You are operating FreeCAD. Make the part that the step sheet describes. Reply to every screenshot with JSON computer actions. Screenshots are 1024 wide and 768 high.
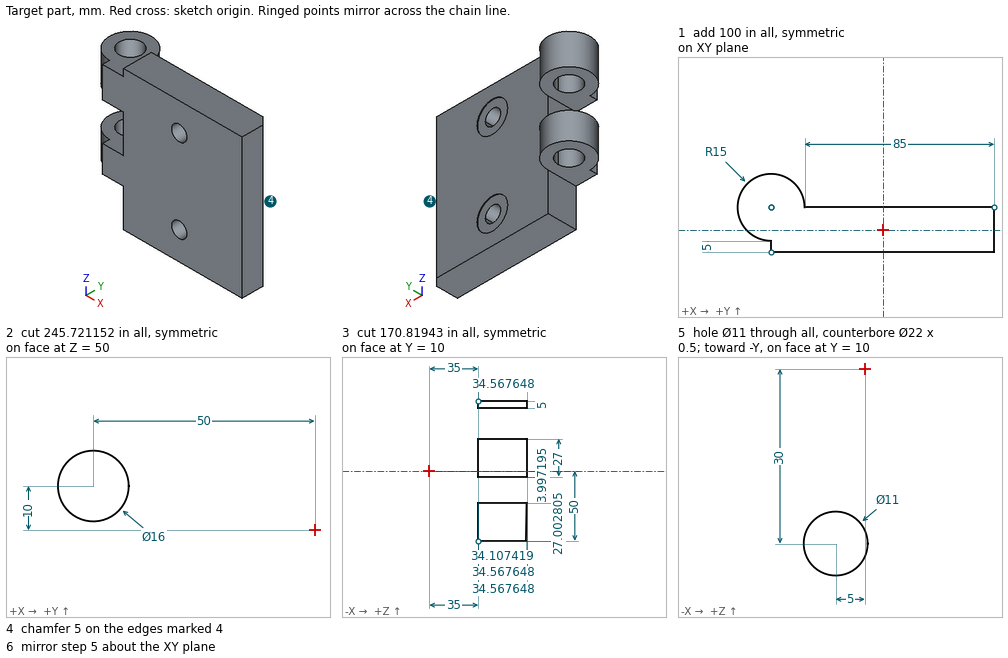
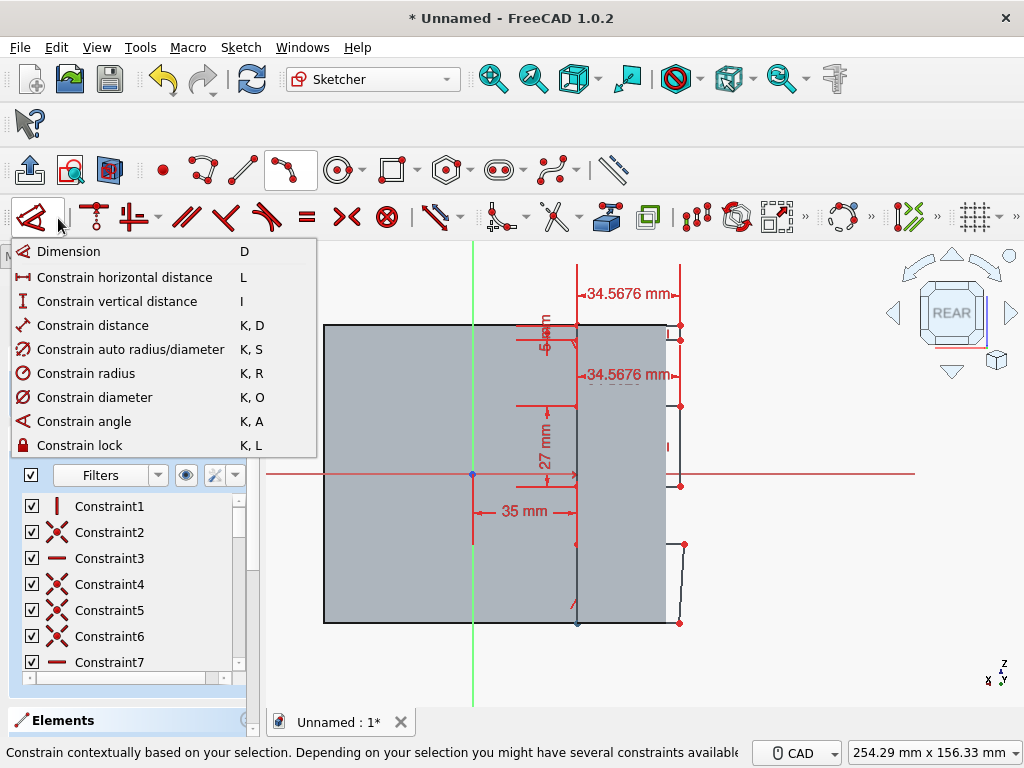
{"action": "left_click", "coordinate": [164, 301]}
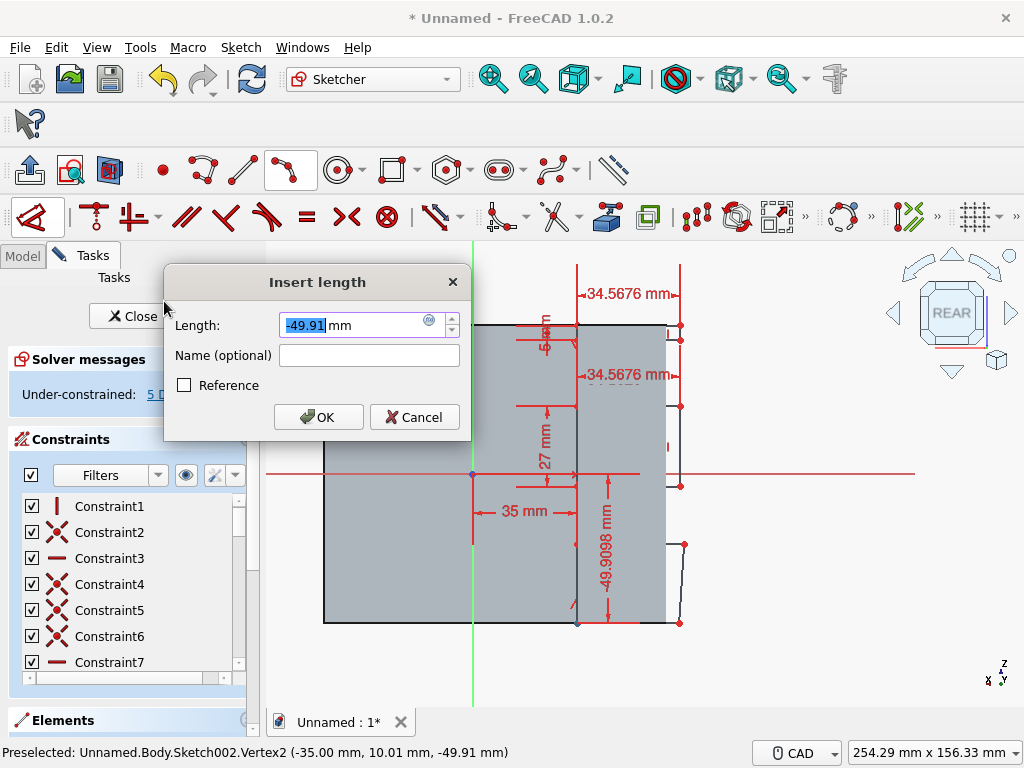
{"action": "type", "text": "-50"}
{"action": "key", "text": "Return"}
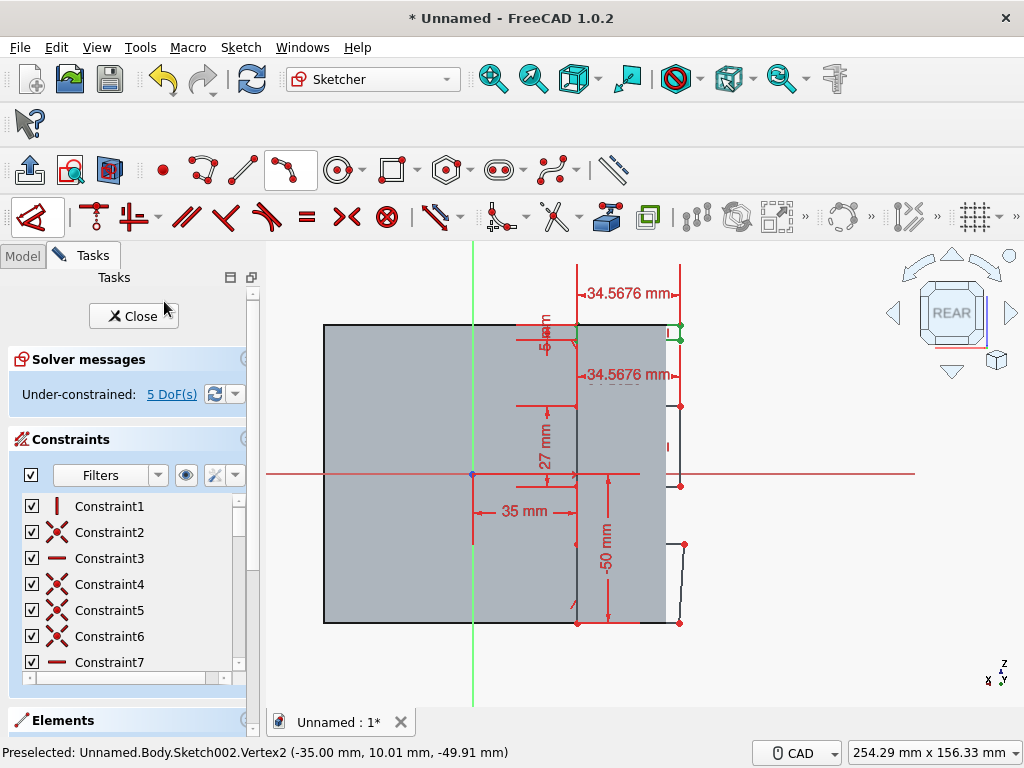
{"action": "left_click", "coordinate": [577, 406]}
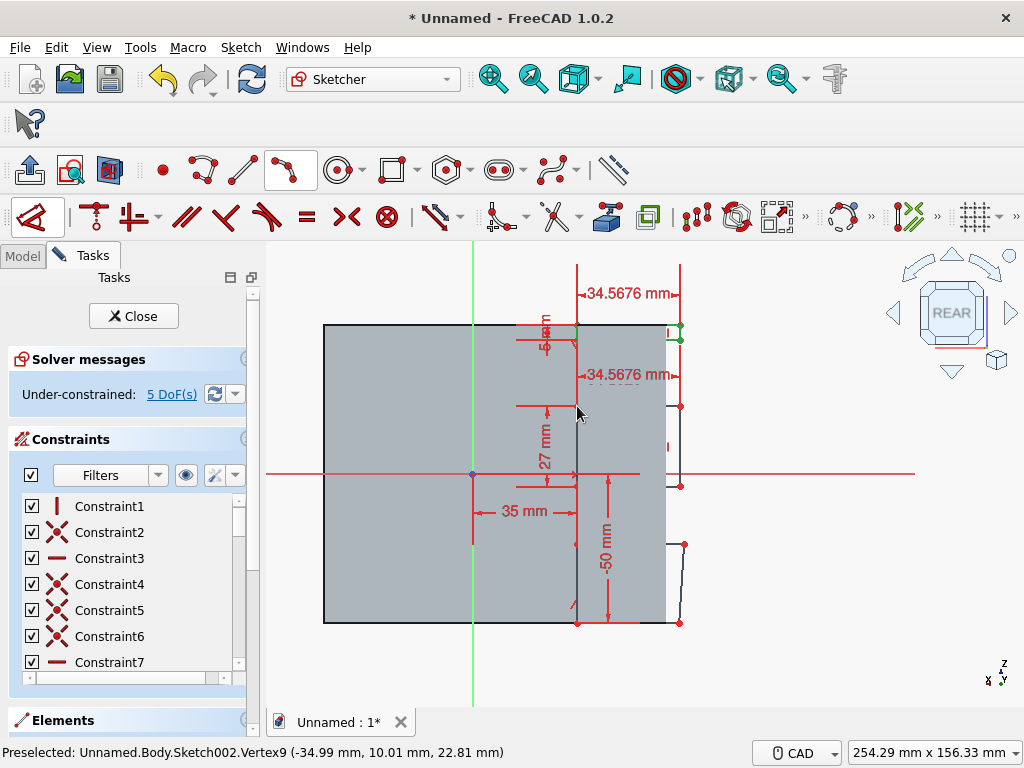
{"action": "key", "text": "l"}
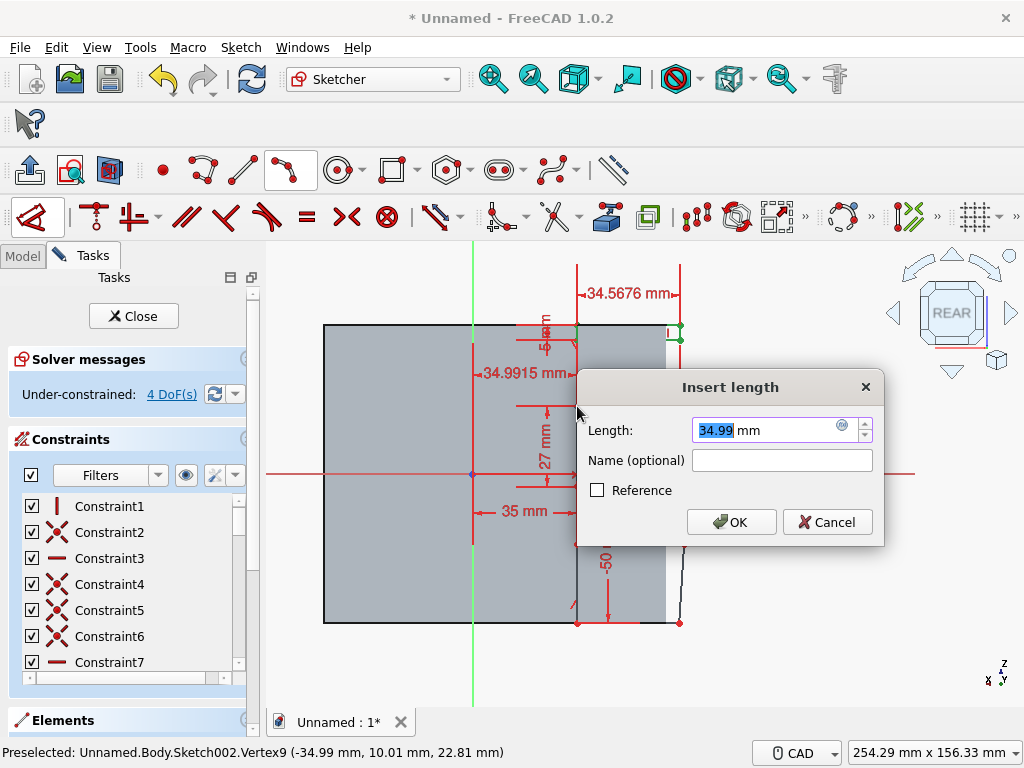
{"action": "type", "text": "35"}
{"action": "key", "text": "Return"}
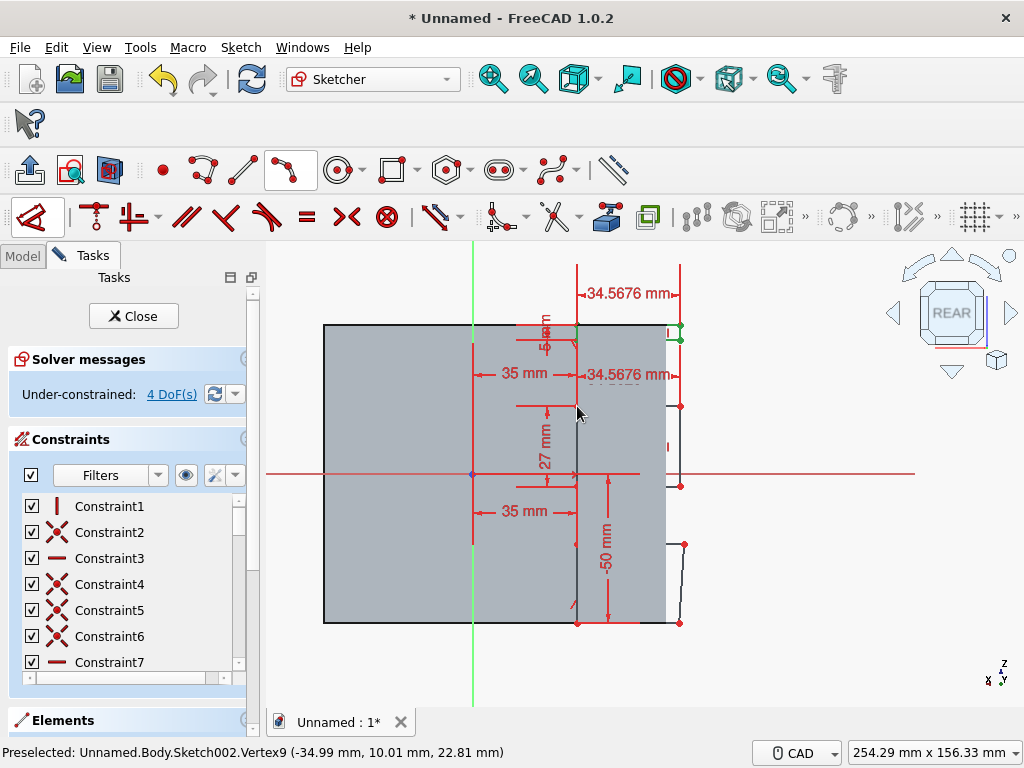
{"action": "left_click", "coordinate": [577, 568]}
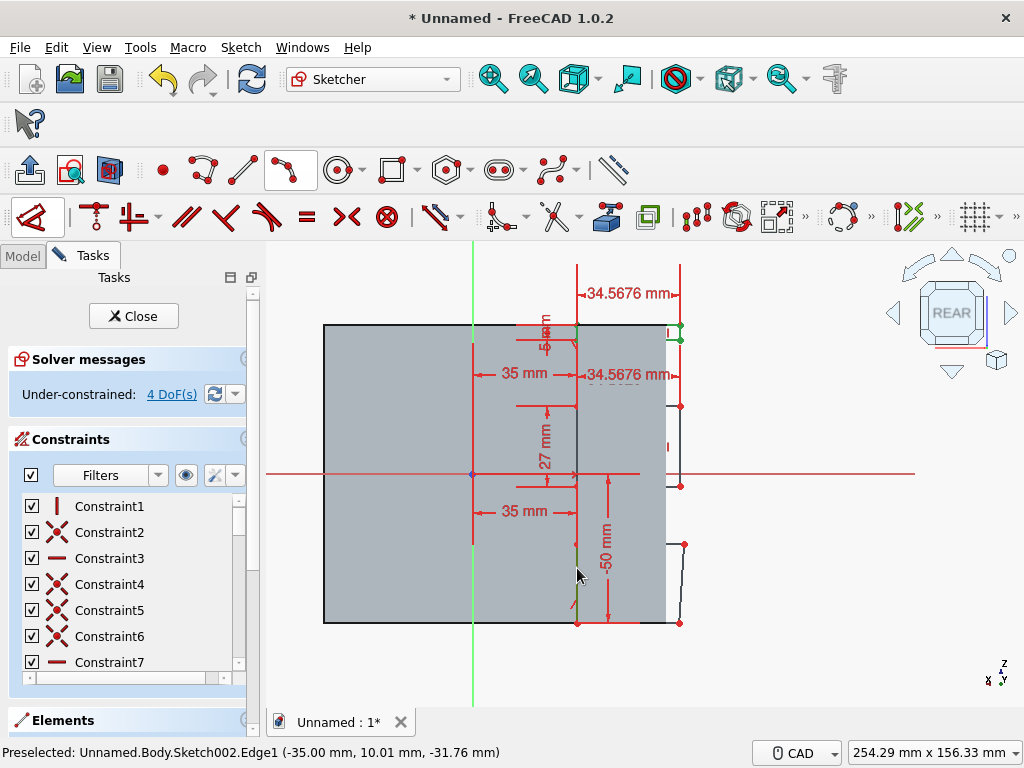
{"action": "key", "text": "i"}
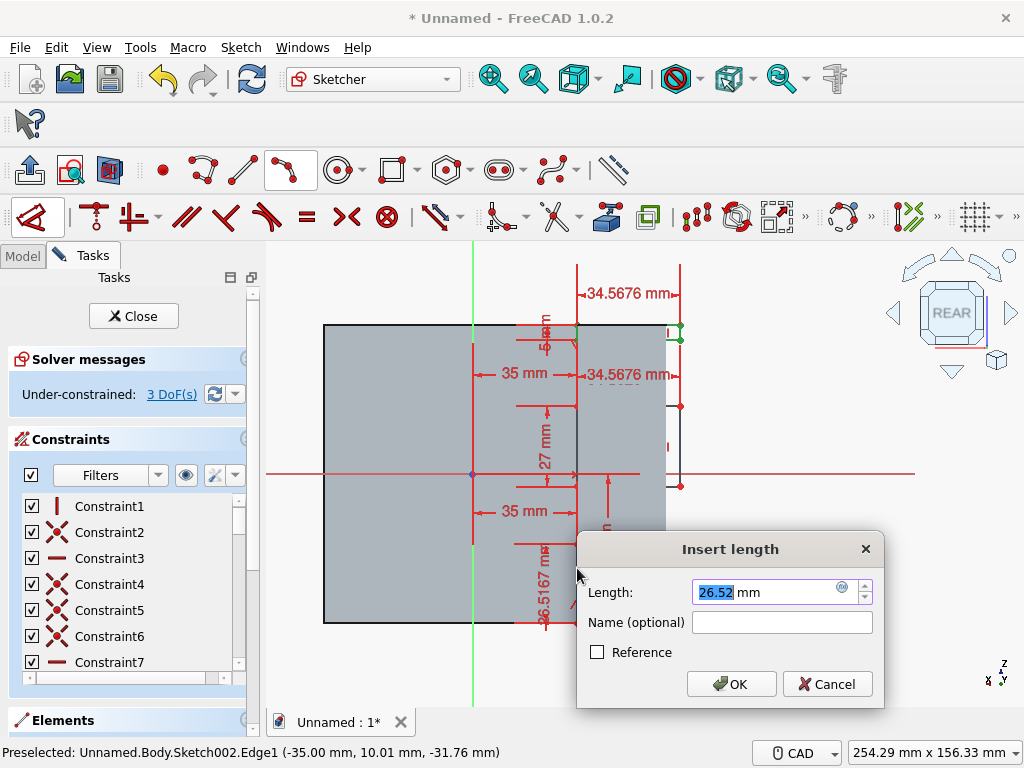
{"action": "type", "text": "27.002805"}
{"action": "key", "text": "Return"}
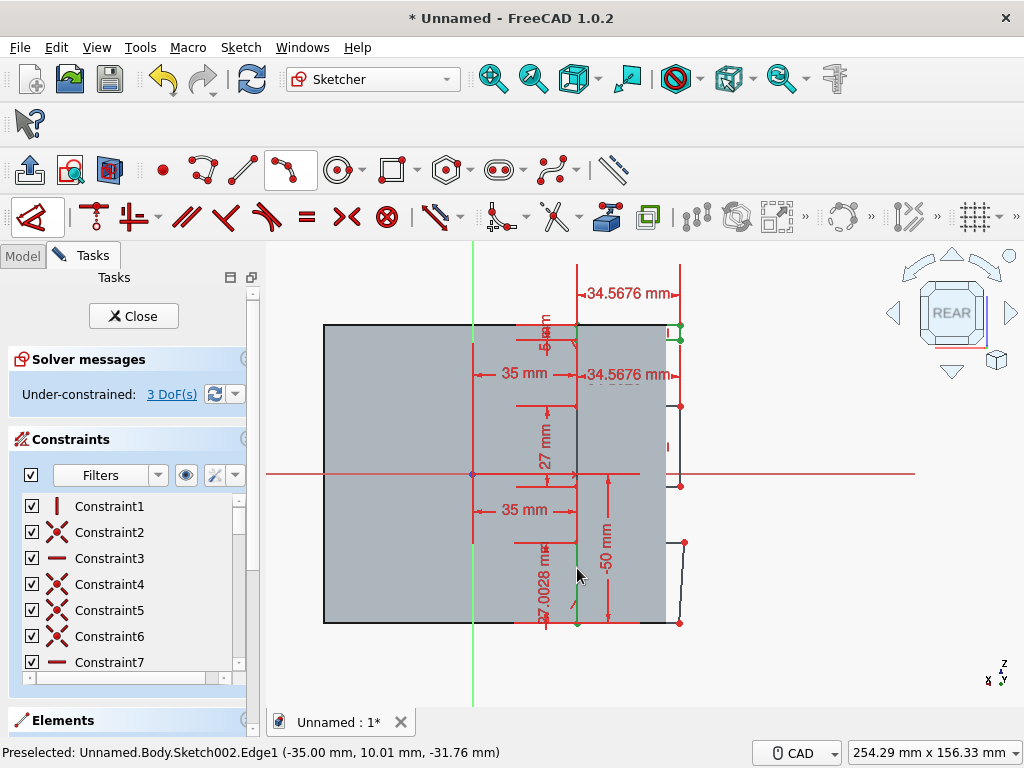
{"action": "left_click", "coordinate": [608, 623]}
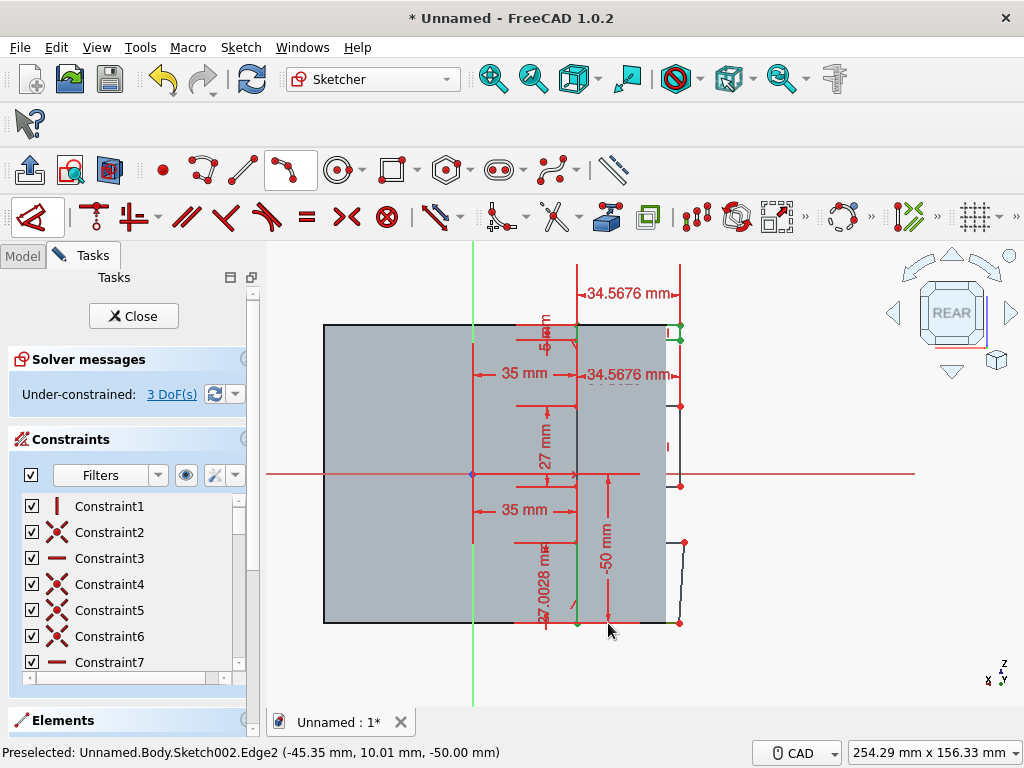
{"action": "left_click", "coordinate": [58, 218]}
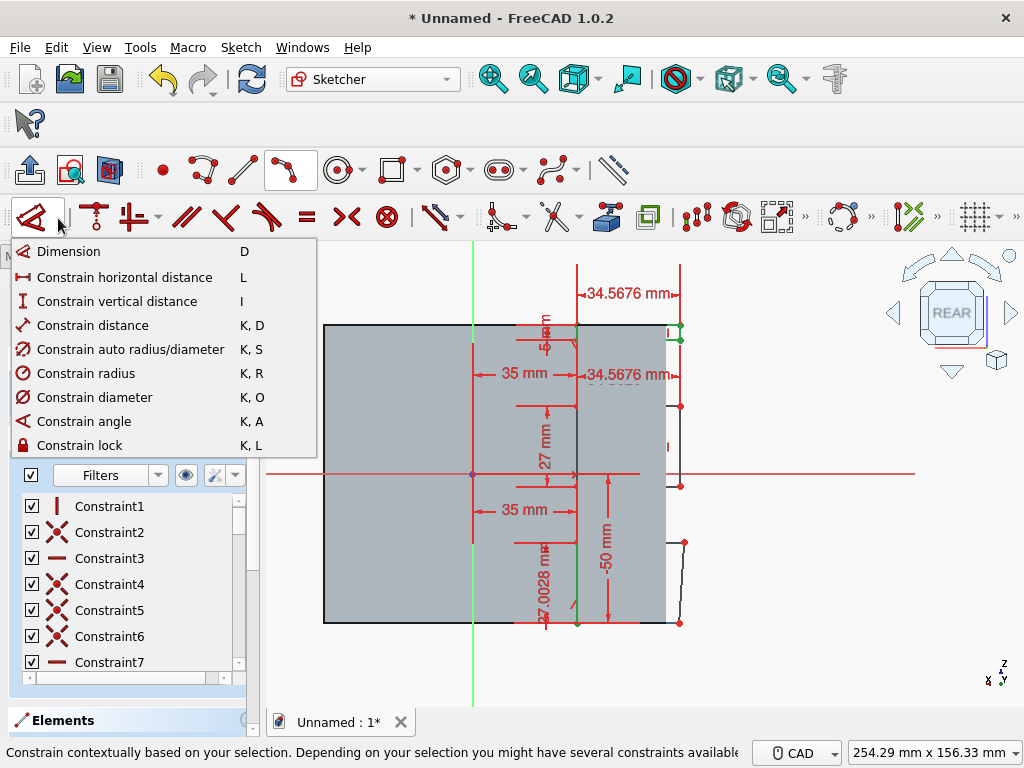
{"action": "left_click", "coordinate": [164, 277]}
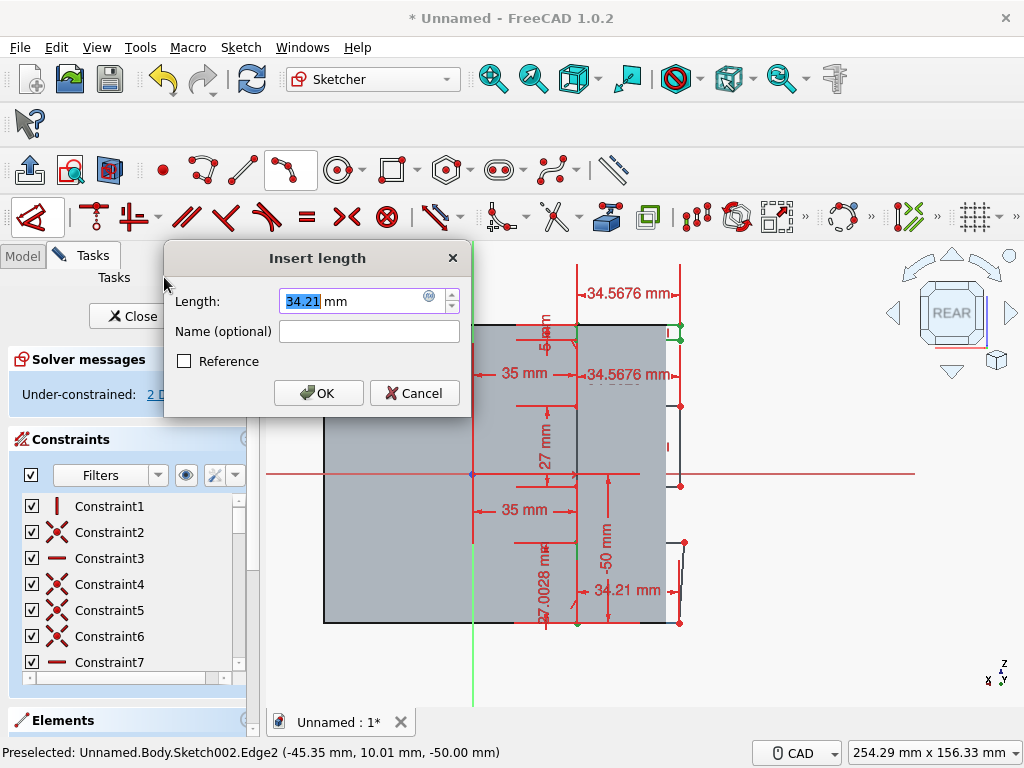
{"action": "type", "text": "34.107419"}
{"action": "key", "text": "Return"}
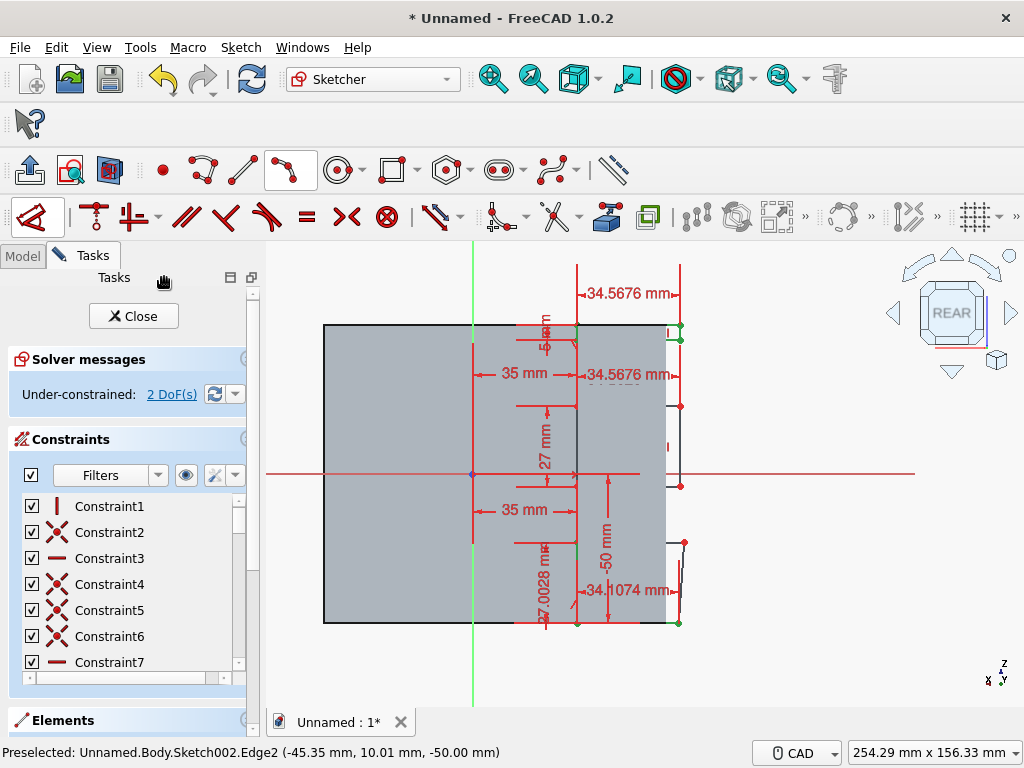
{"action": "left_click", "coordinate": [652, 543]}